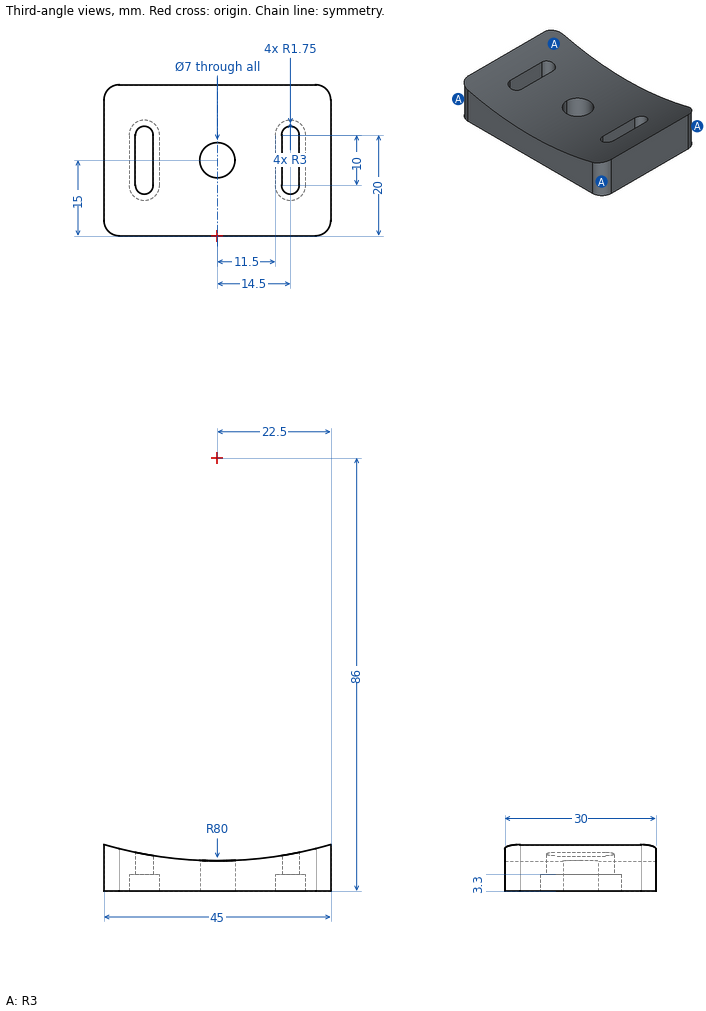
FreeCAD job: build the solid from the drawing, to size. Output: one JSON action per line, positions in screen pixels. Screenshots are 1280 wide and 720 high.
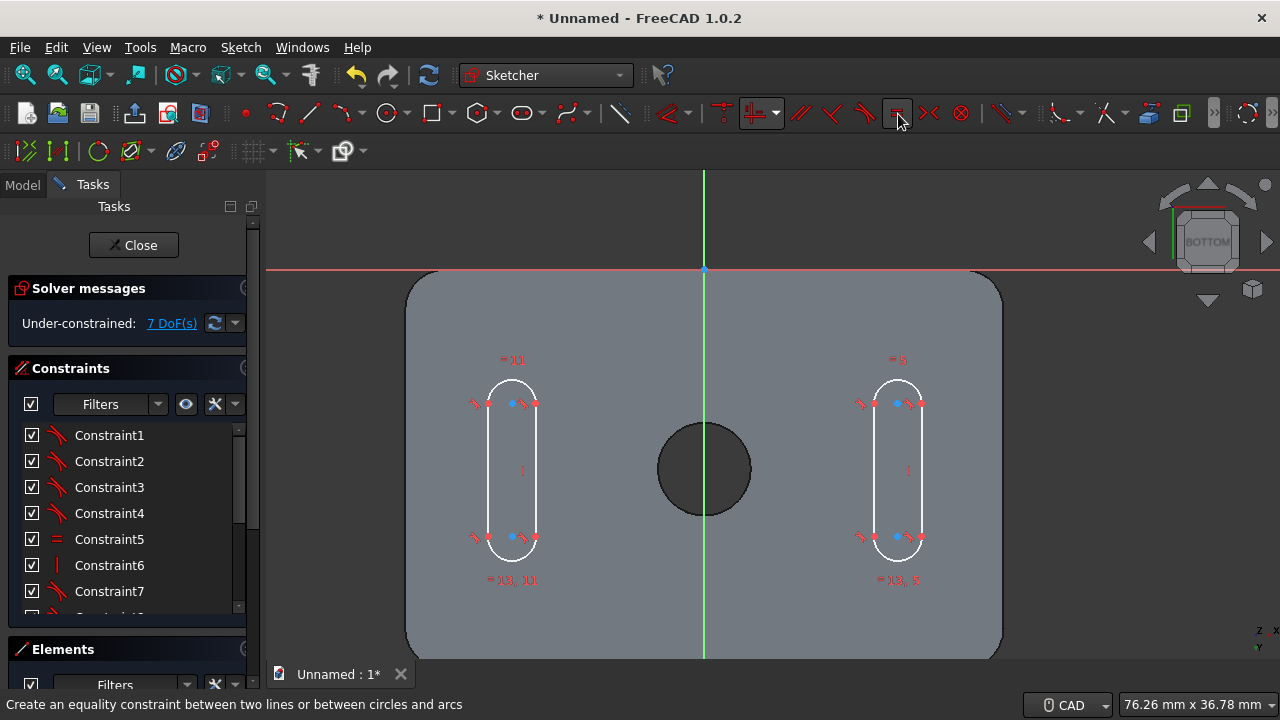
{"action": "left_click", "coordinate": [898, 537]}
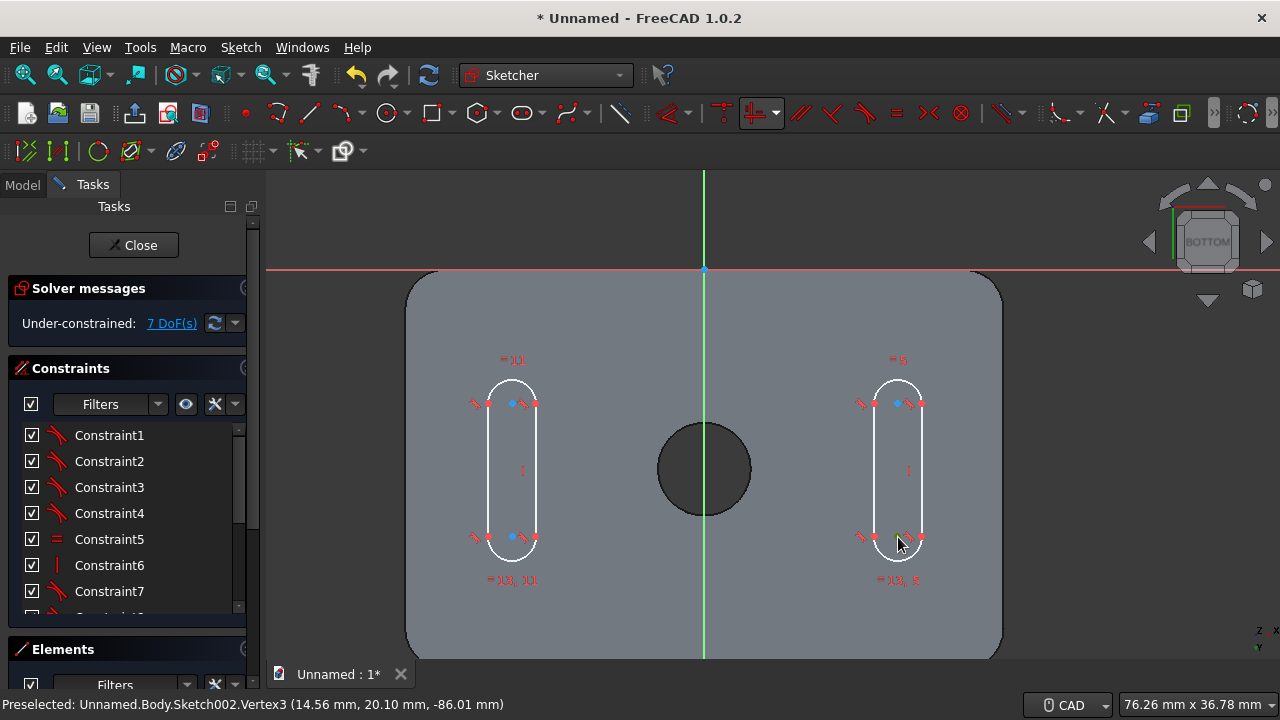
{"action": "left_click", "coordinate": [512, 537]}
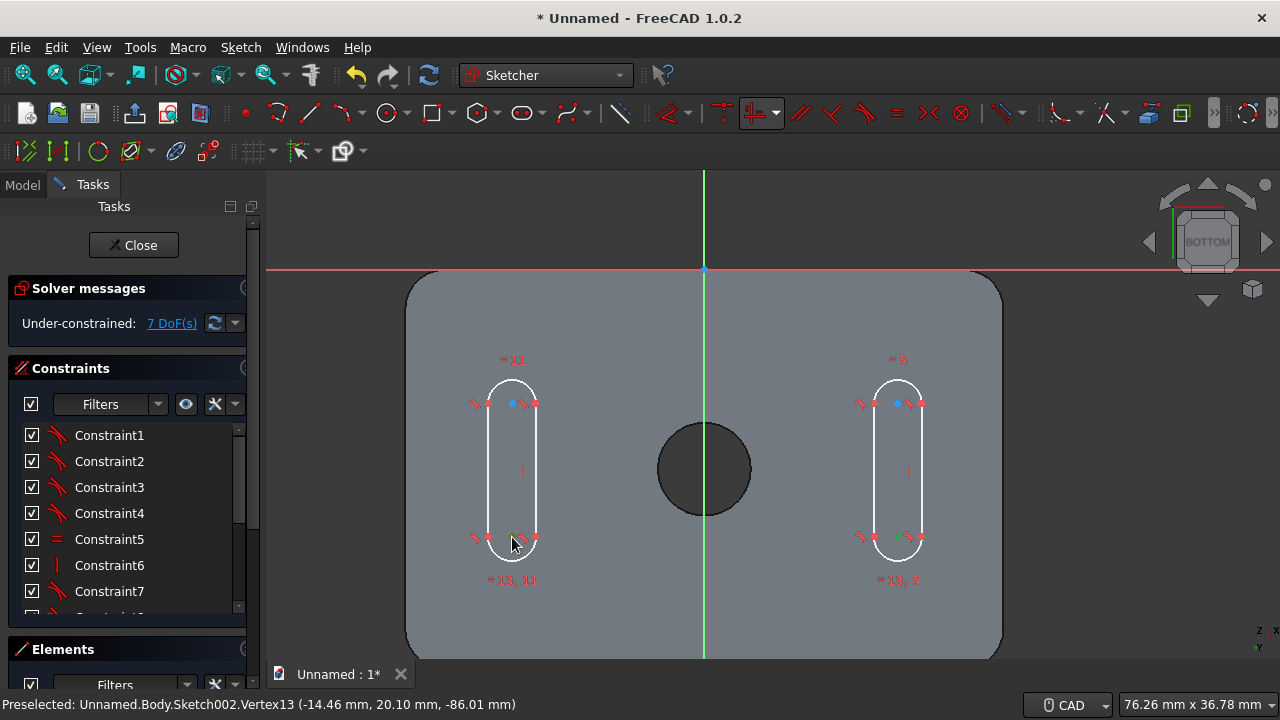
{"action": "left_click", "coordinate": [704, 600]}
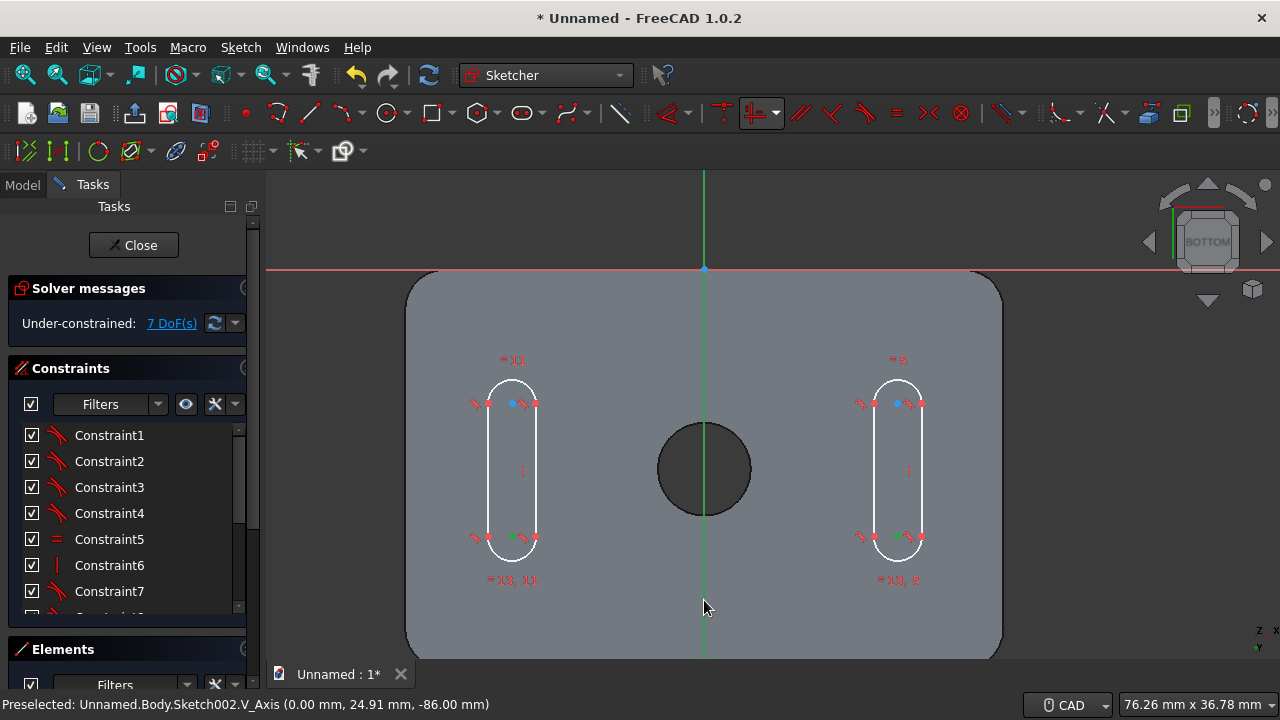
{"action": "left_click", "coordinate": [930, 114]}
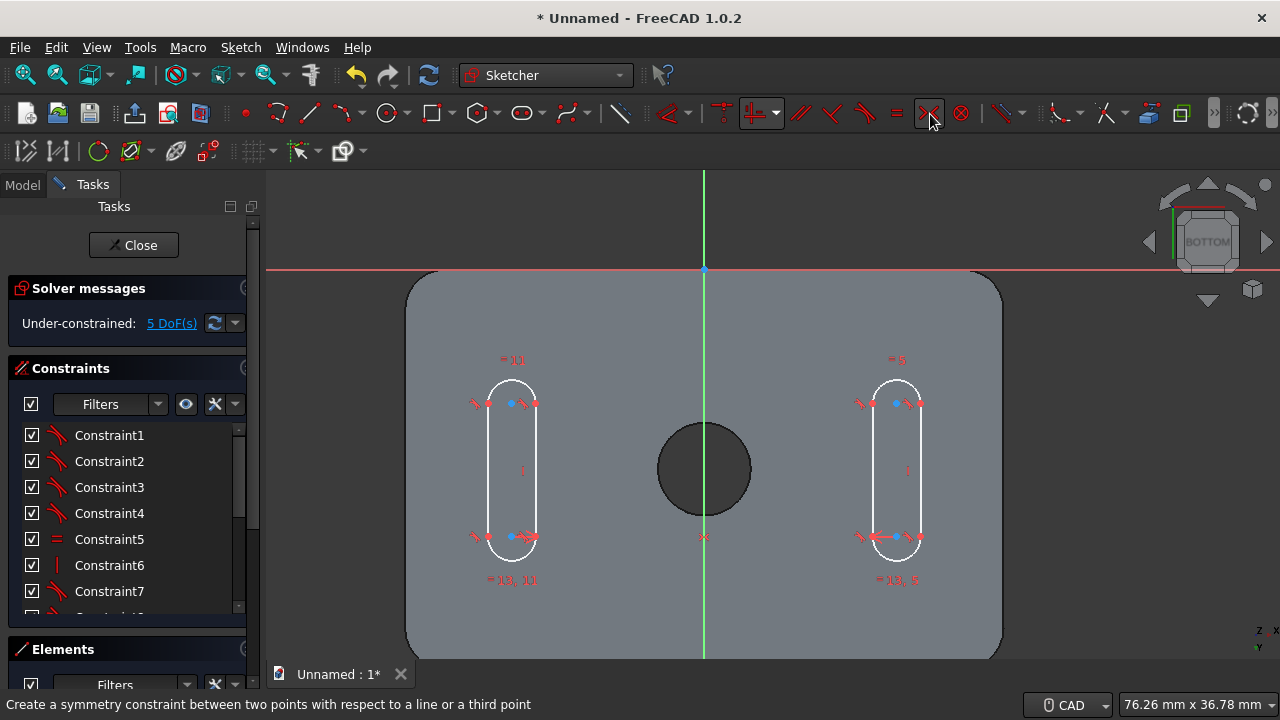
{"action": "left_click", "coordinate": [668, 114]}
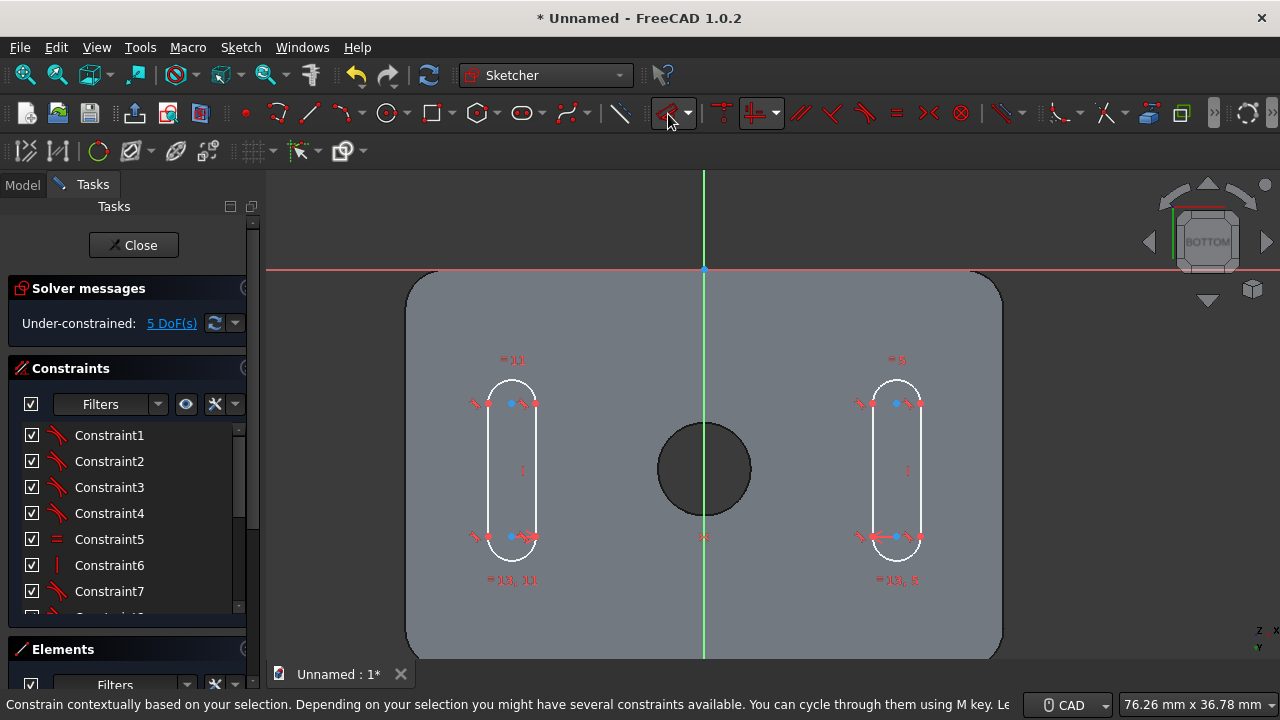
{"action": "scroll", "coordinate": [883, 556], "scroll_direction": "up", "scroll_amount": 3}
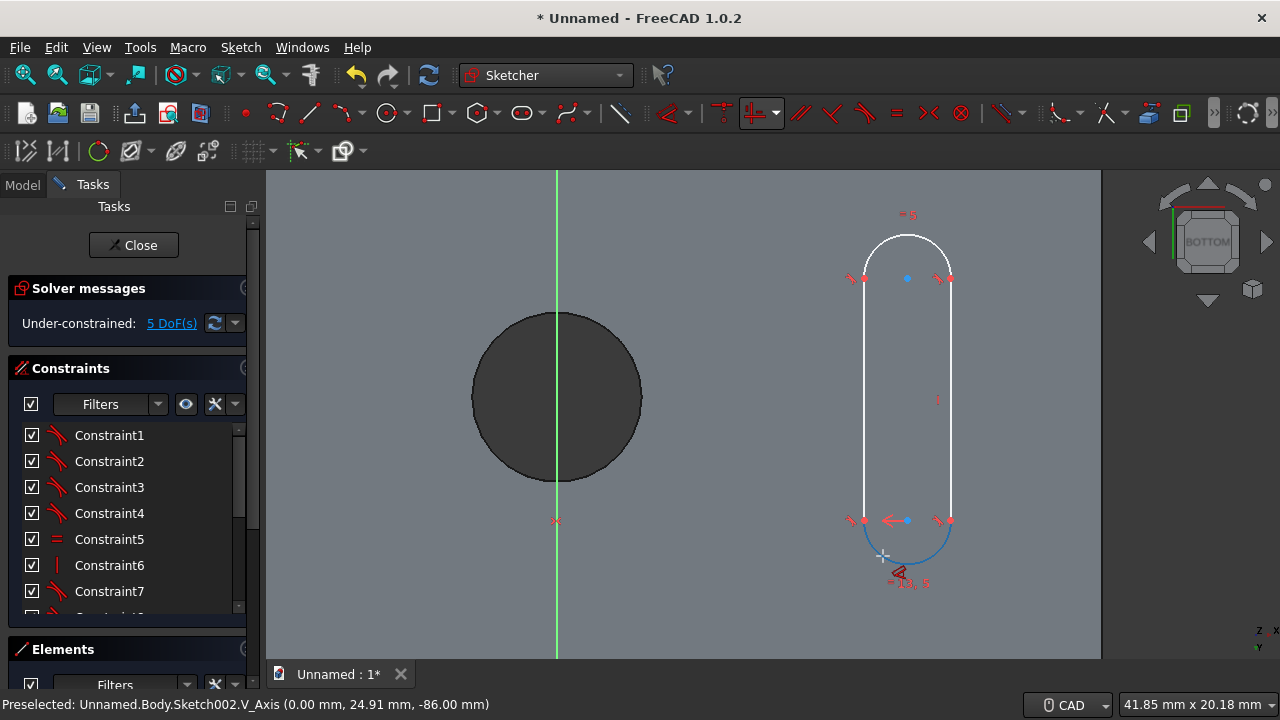
{"action": "left_click", "coordinate": [882, 556]}
{"action": "left_click", "coordinate": [863, 582]}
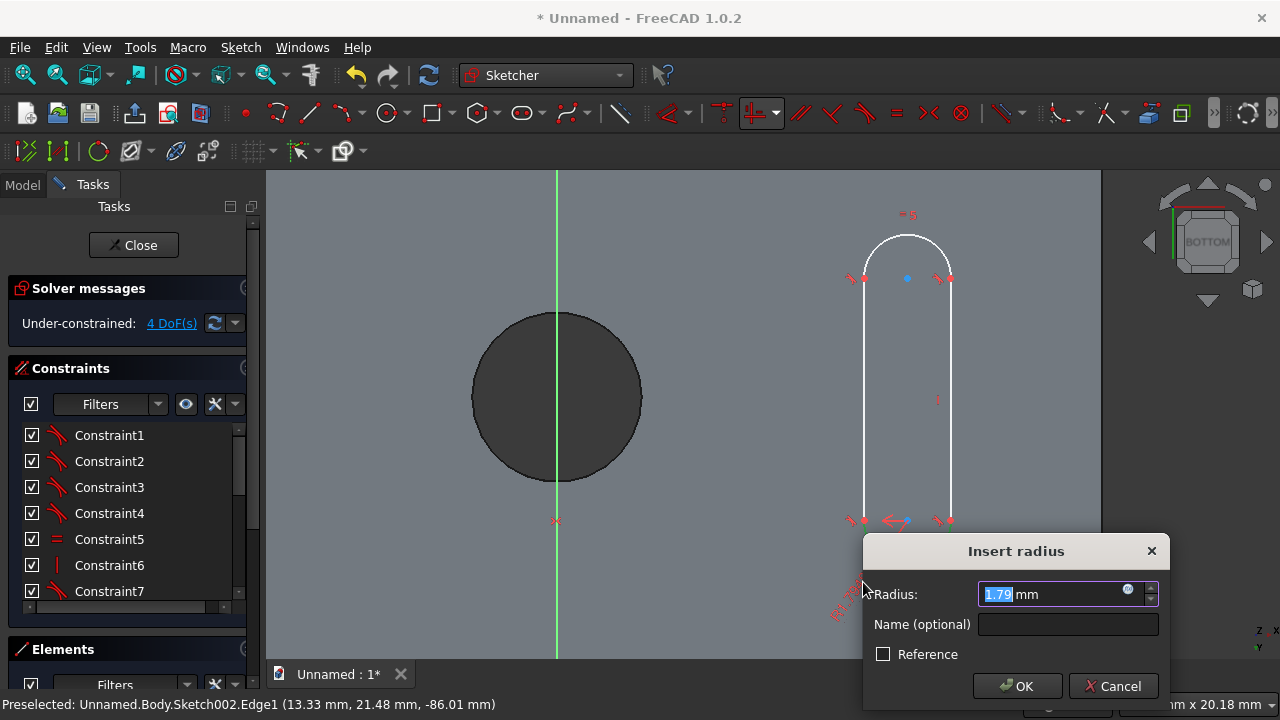
{"action": "type", "text": "1.75"}
{"action": "key", "text": "Return"}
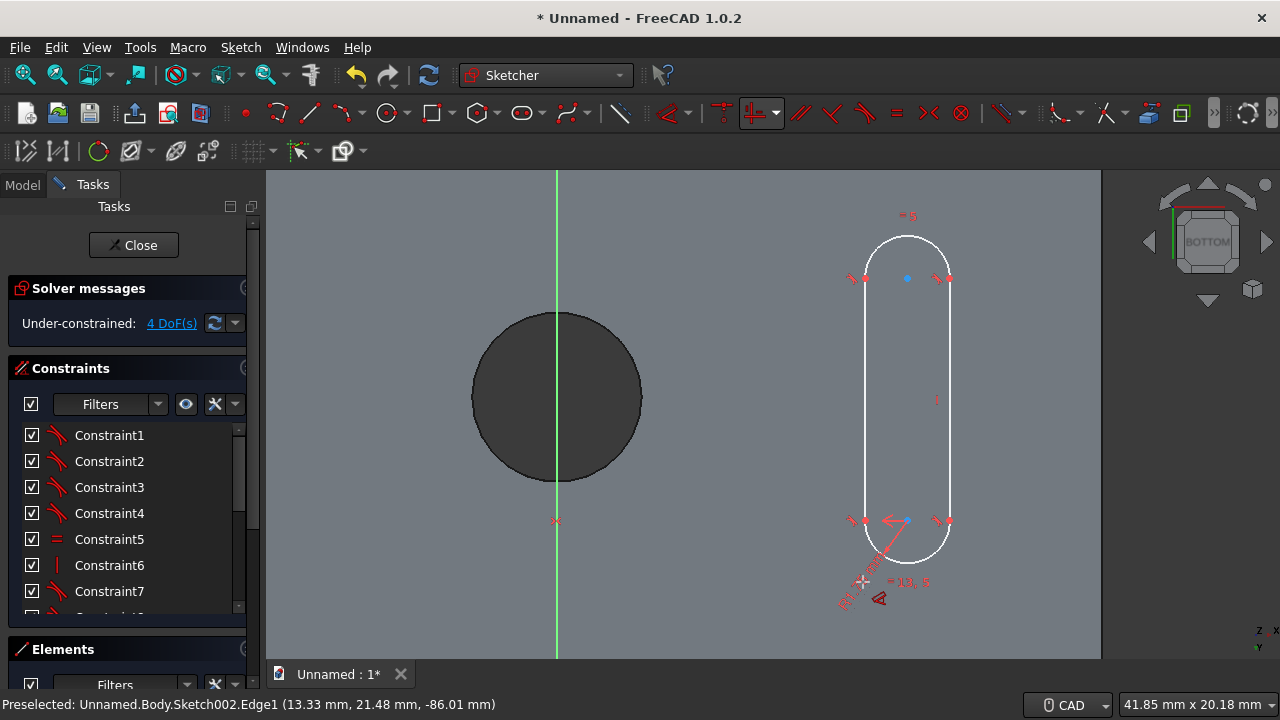
{"action": "left_click", "coordinate": [865, 448]}
{"action": "left_click", "coordinate": [899, 400]}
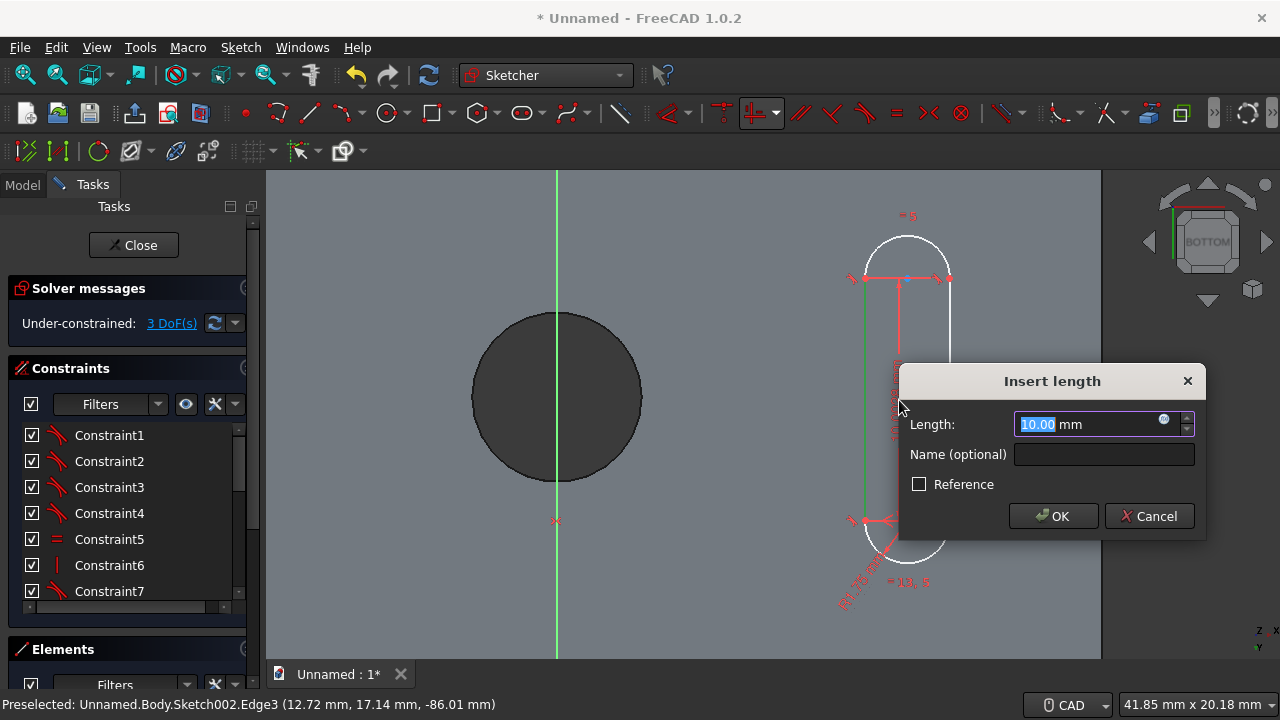
{"action": "type", "text": "10"}
{"action": "key", "text": "Return"}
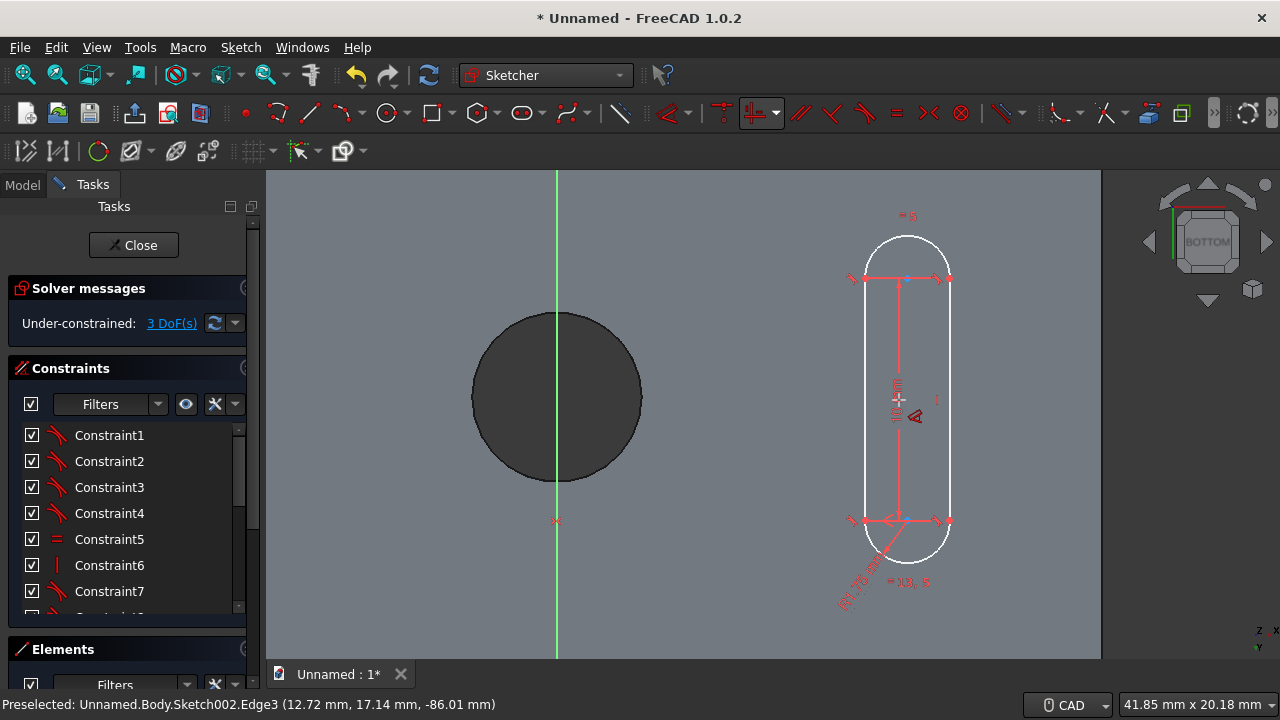
{"action": "scroll", "coordinate": [884, 557], "scroll_direction": "down", "scroll_amount": 3}